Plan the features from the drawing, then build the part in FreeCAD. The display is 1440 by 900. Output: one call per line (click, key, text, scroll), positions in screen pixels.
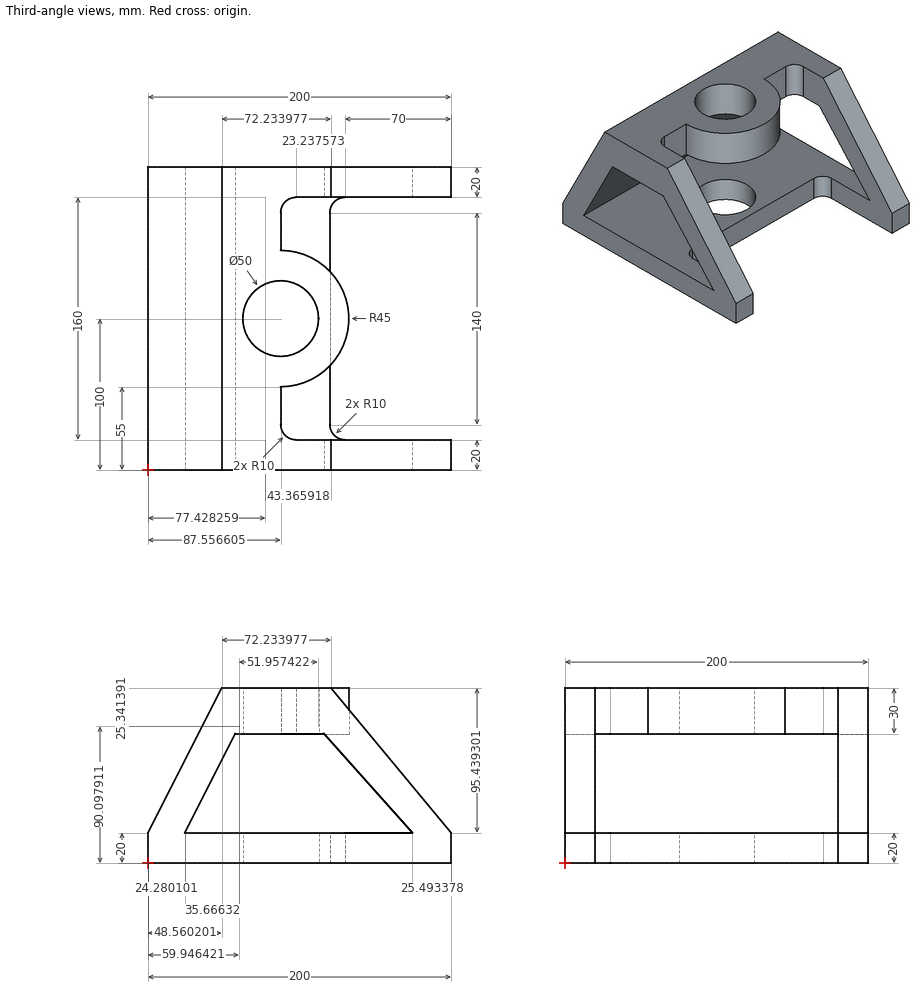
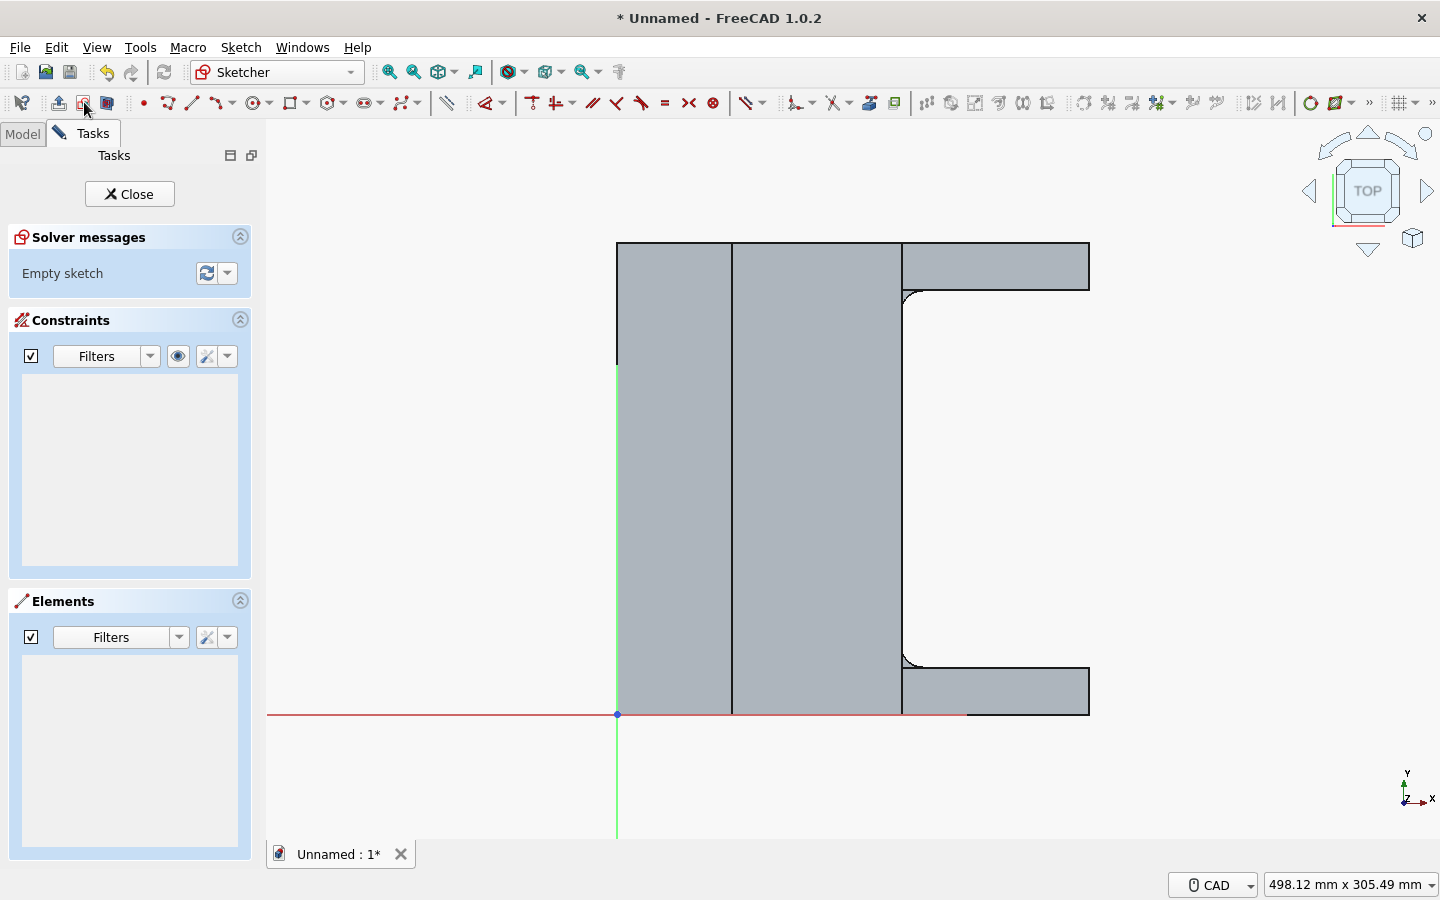
click(290, 104)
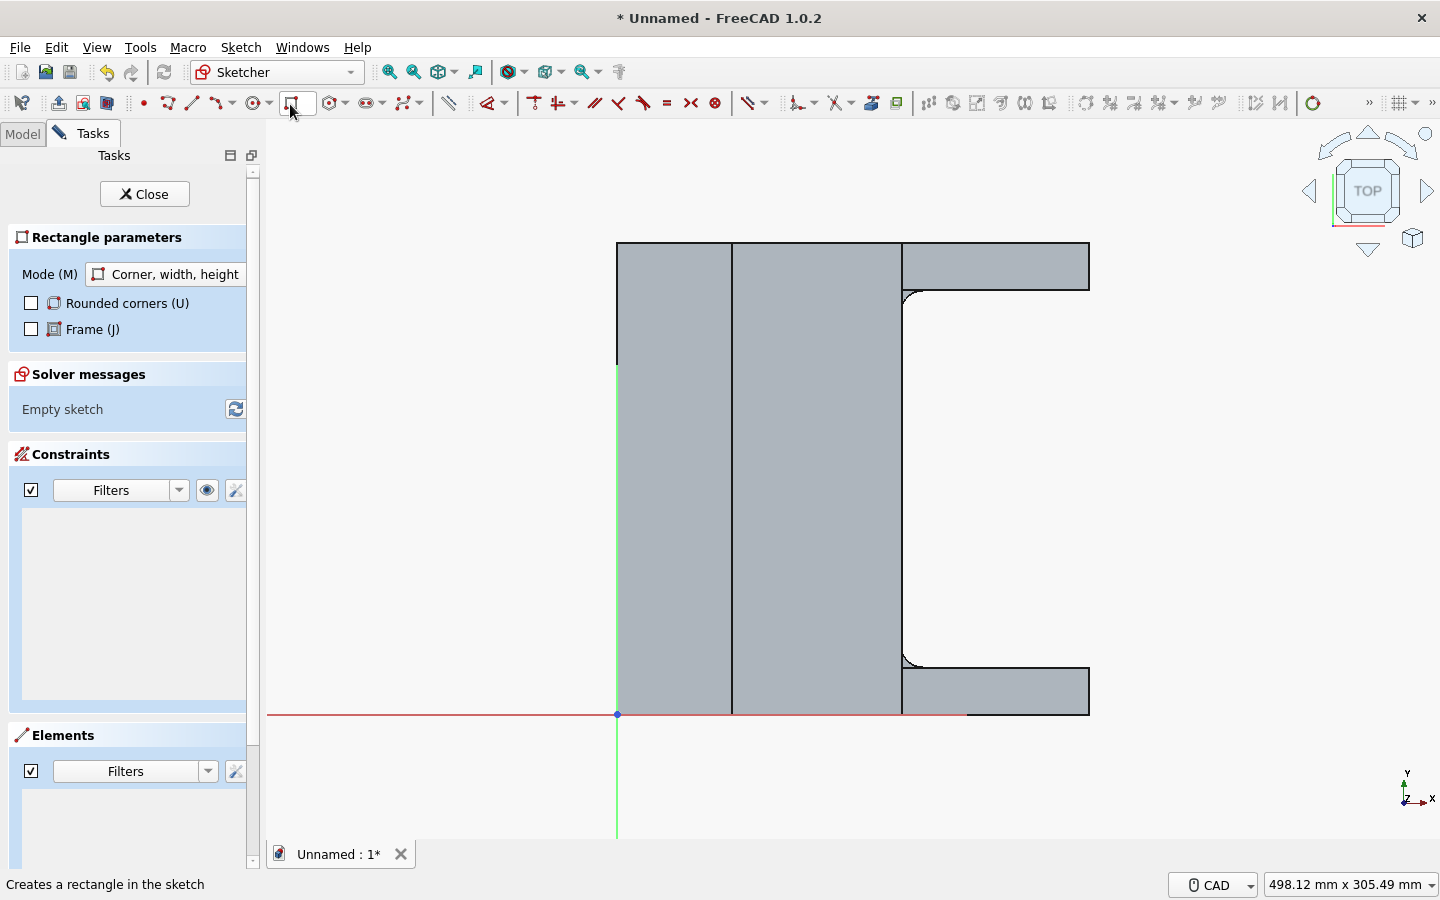
click(800, 290)
click(902, 668)
key(Escape)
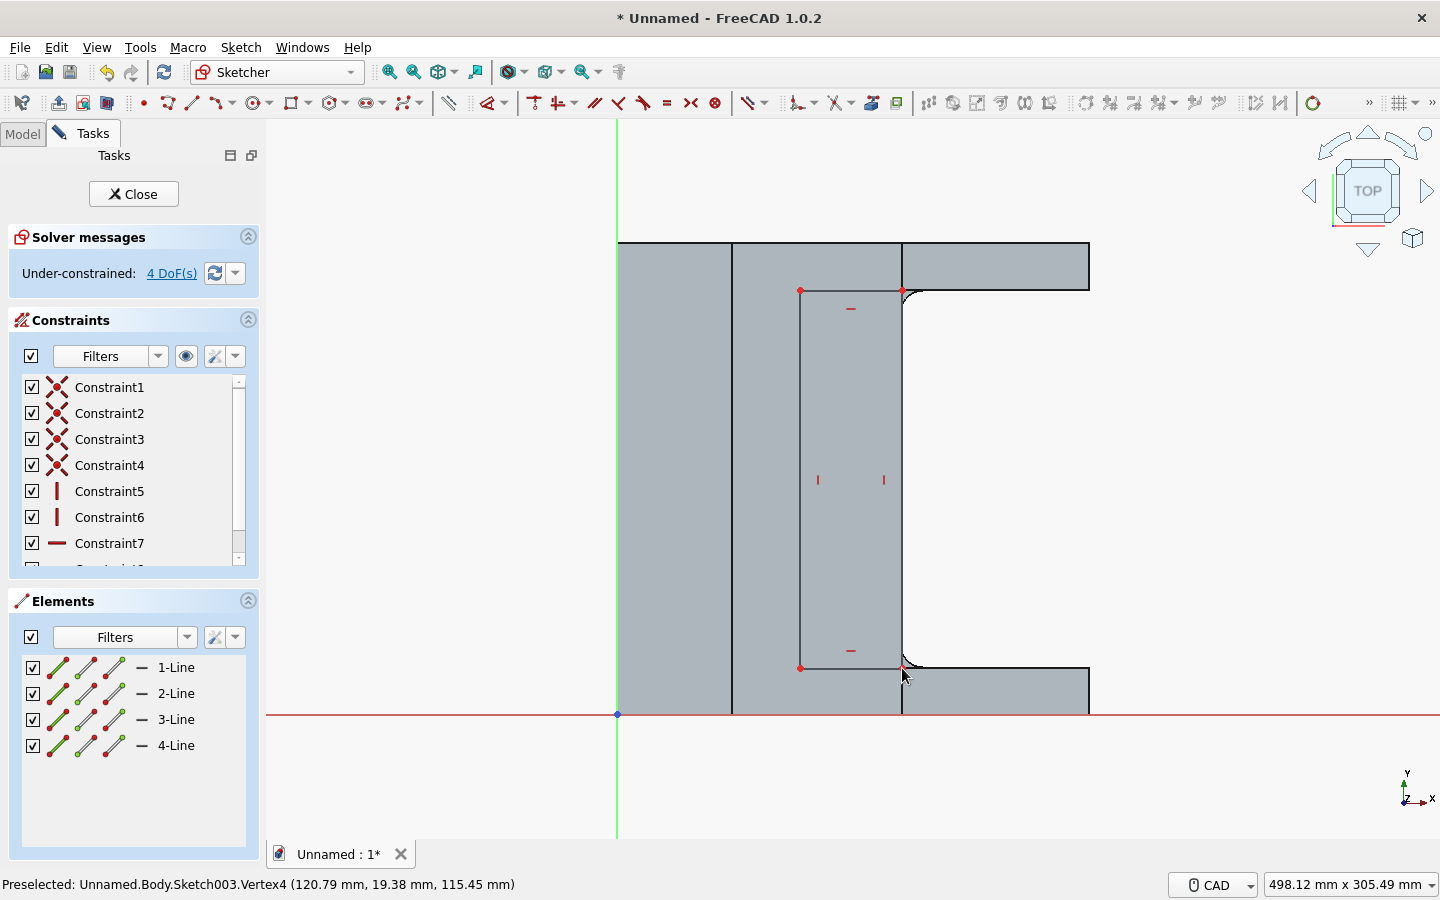
click(488, 104)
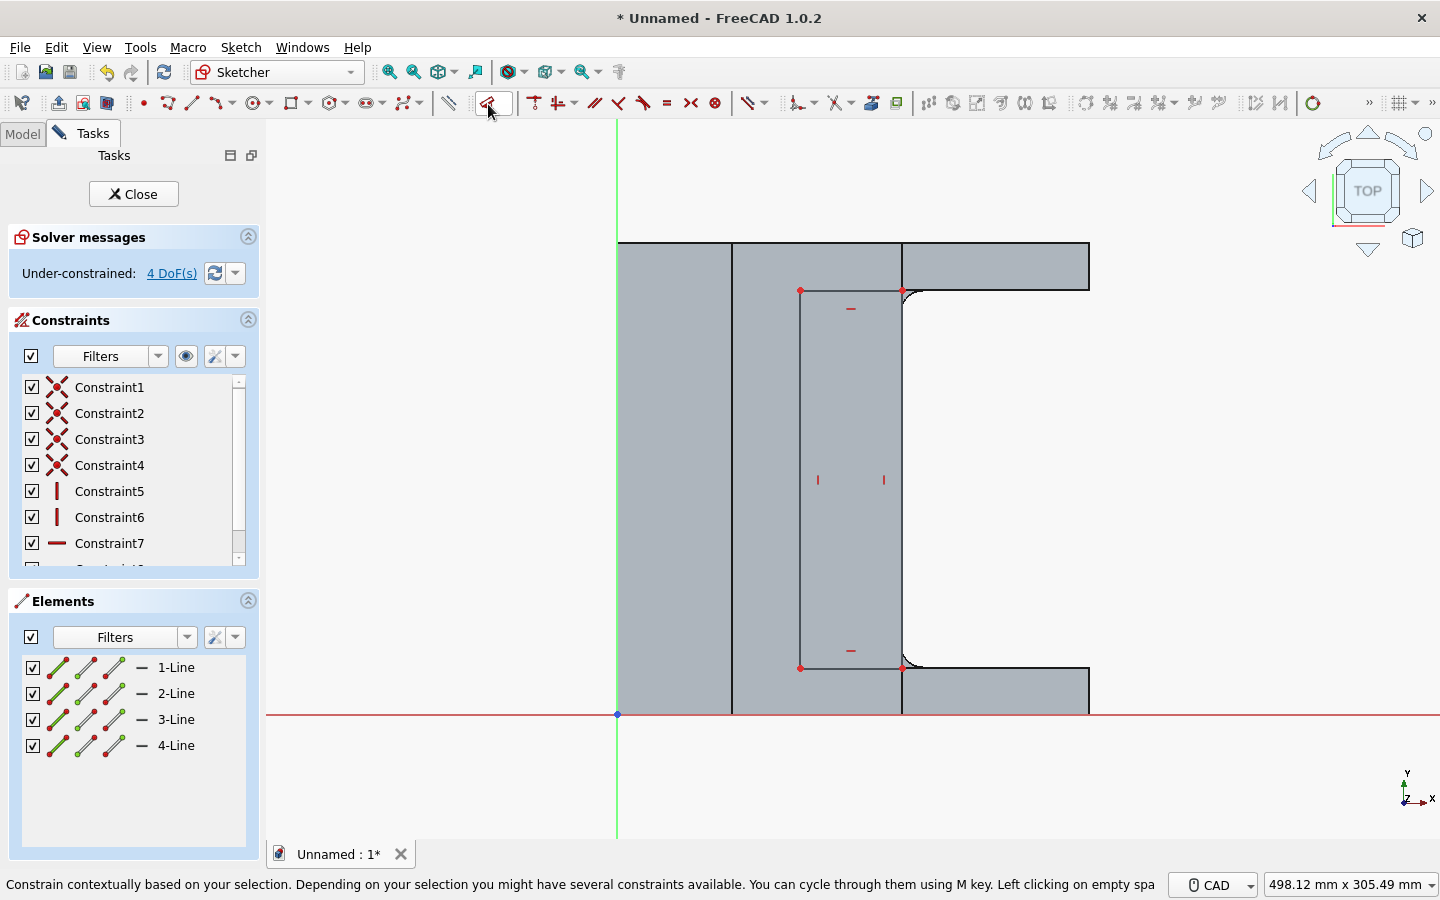
click(800, 404)
click(834, 480)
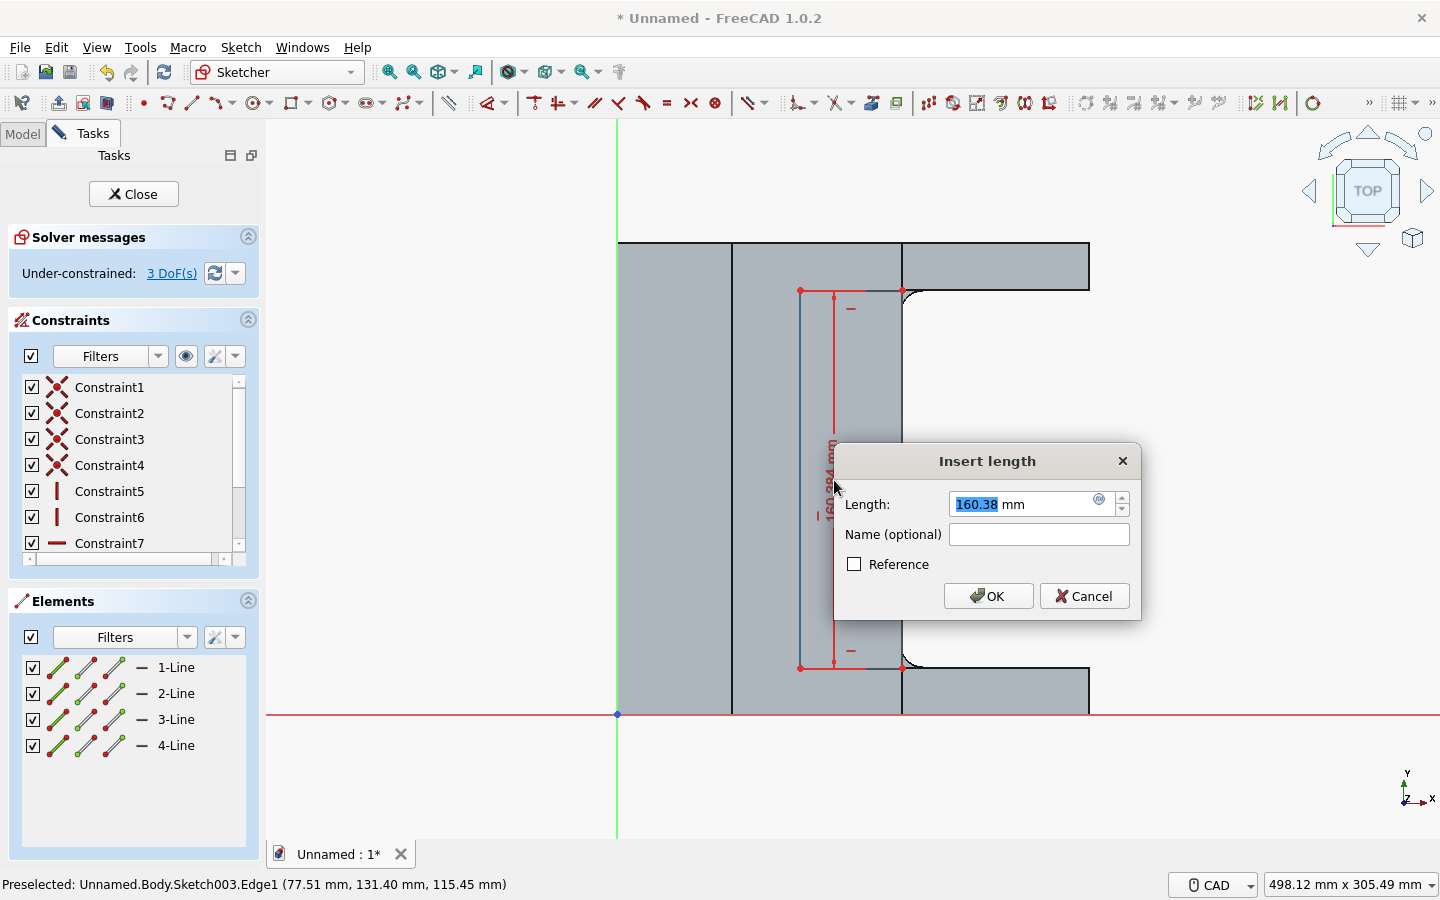
text(160)
key(Return)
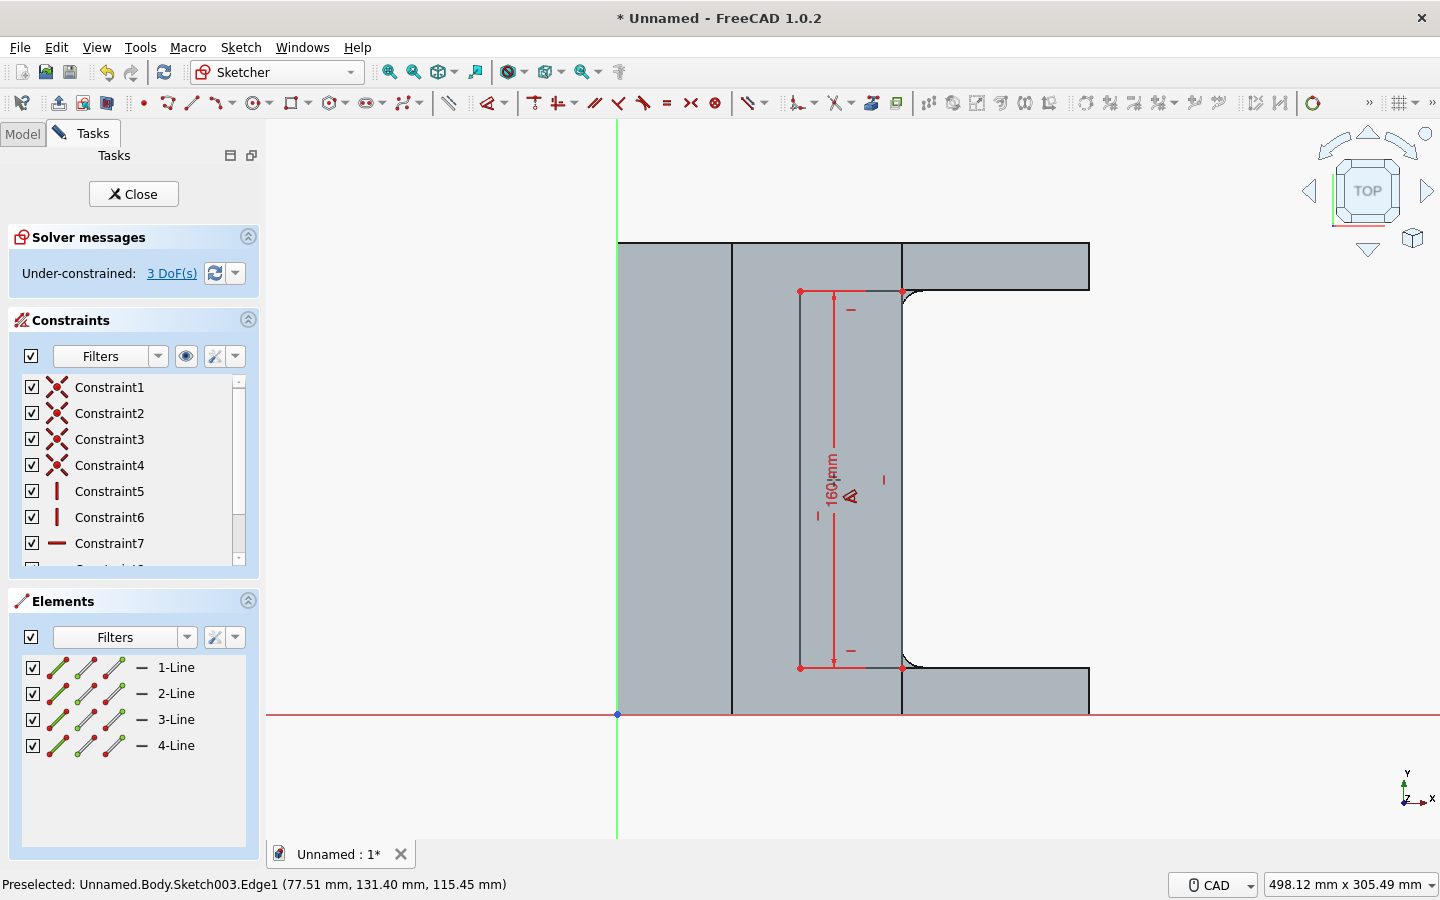
click(800, 668)
click(583, 691)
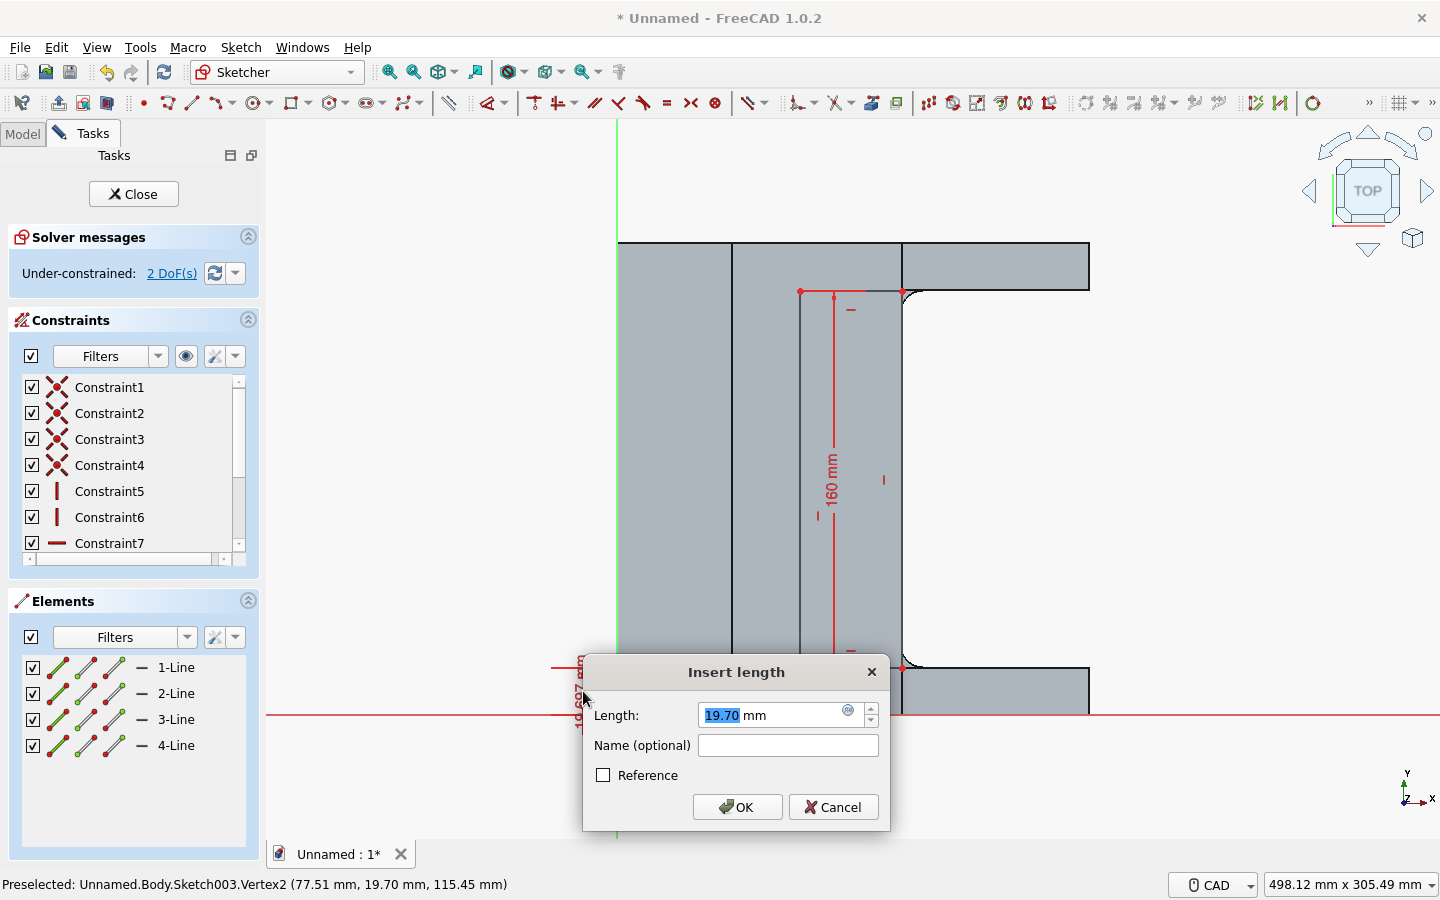
text(20)
key(Return)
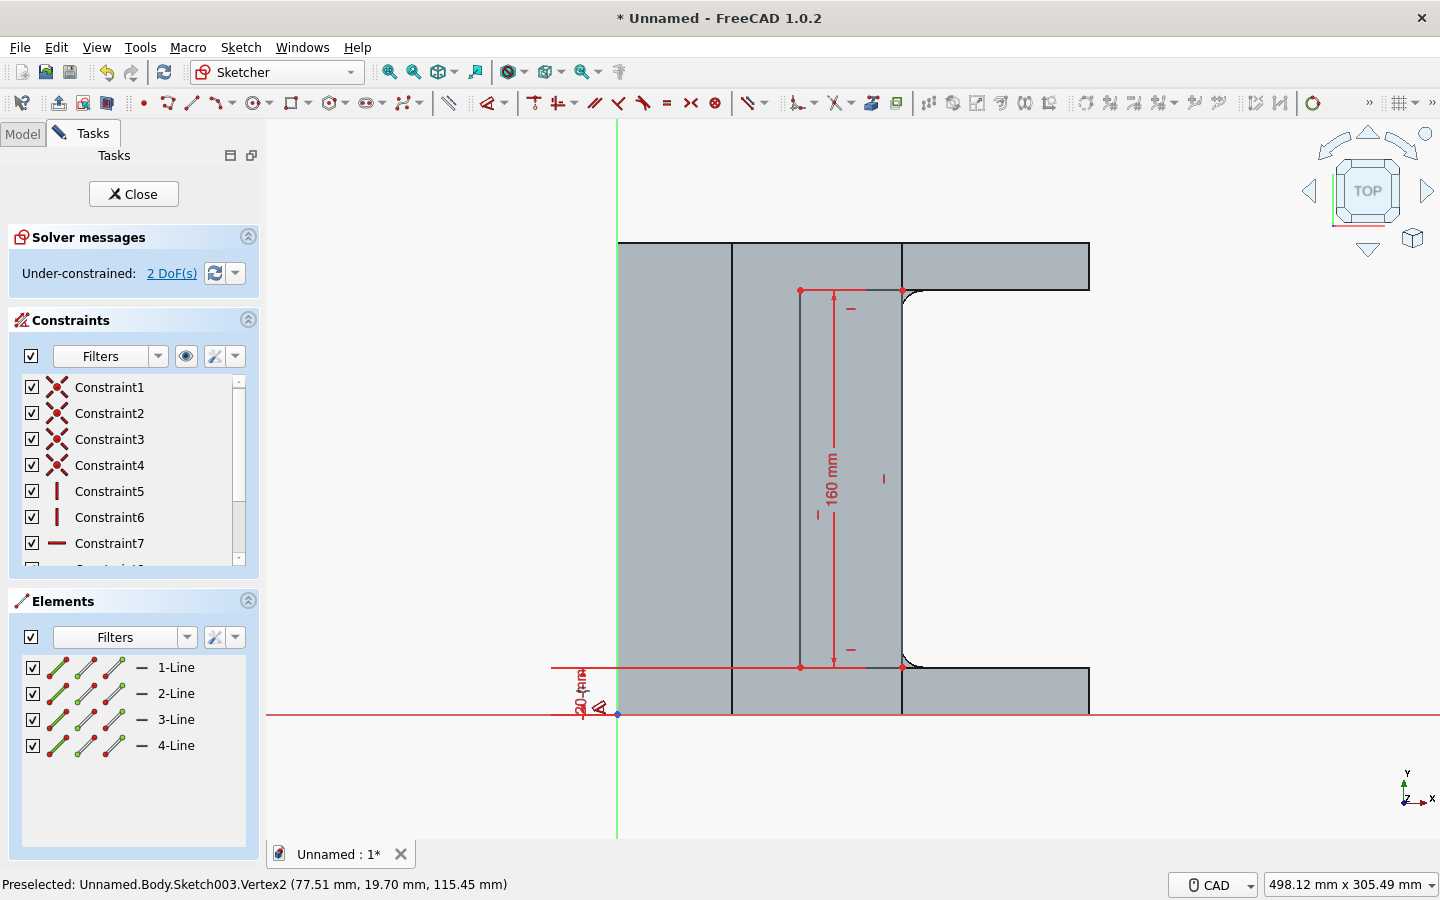
click(831, 668)
click(851, 702)